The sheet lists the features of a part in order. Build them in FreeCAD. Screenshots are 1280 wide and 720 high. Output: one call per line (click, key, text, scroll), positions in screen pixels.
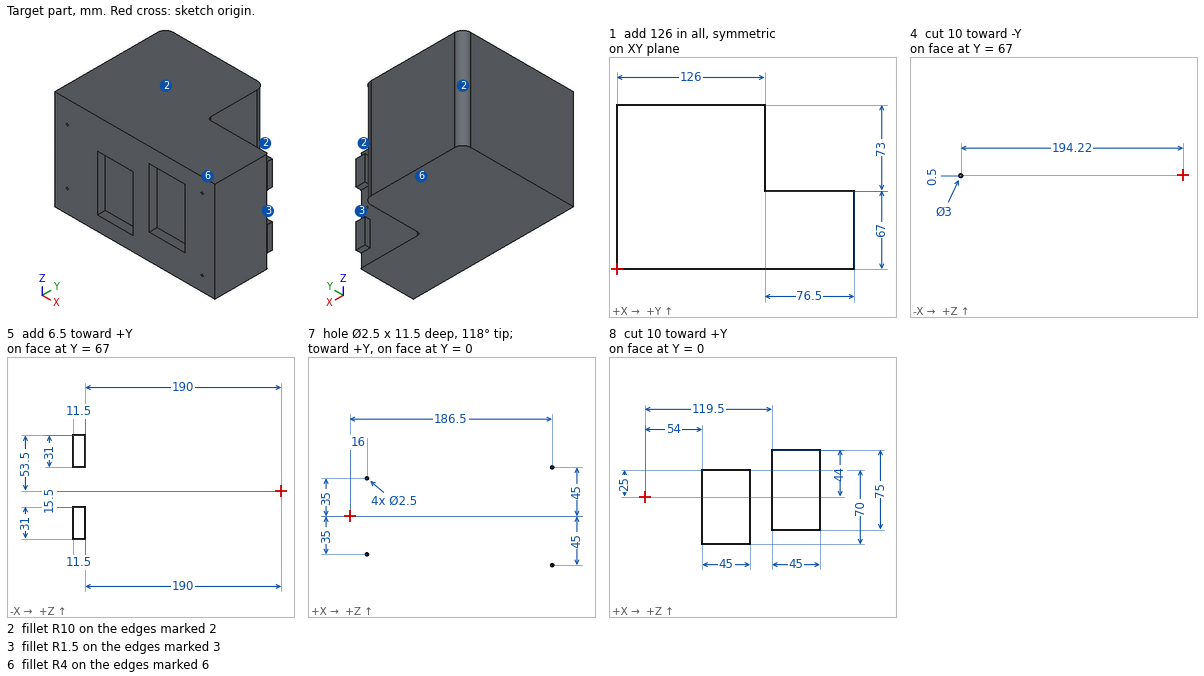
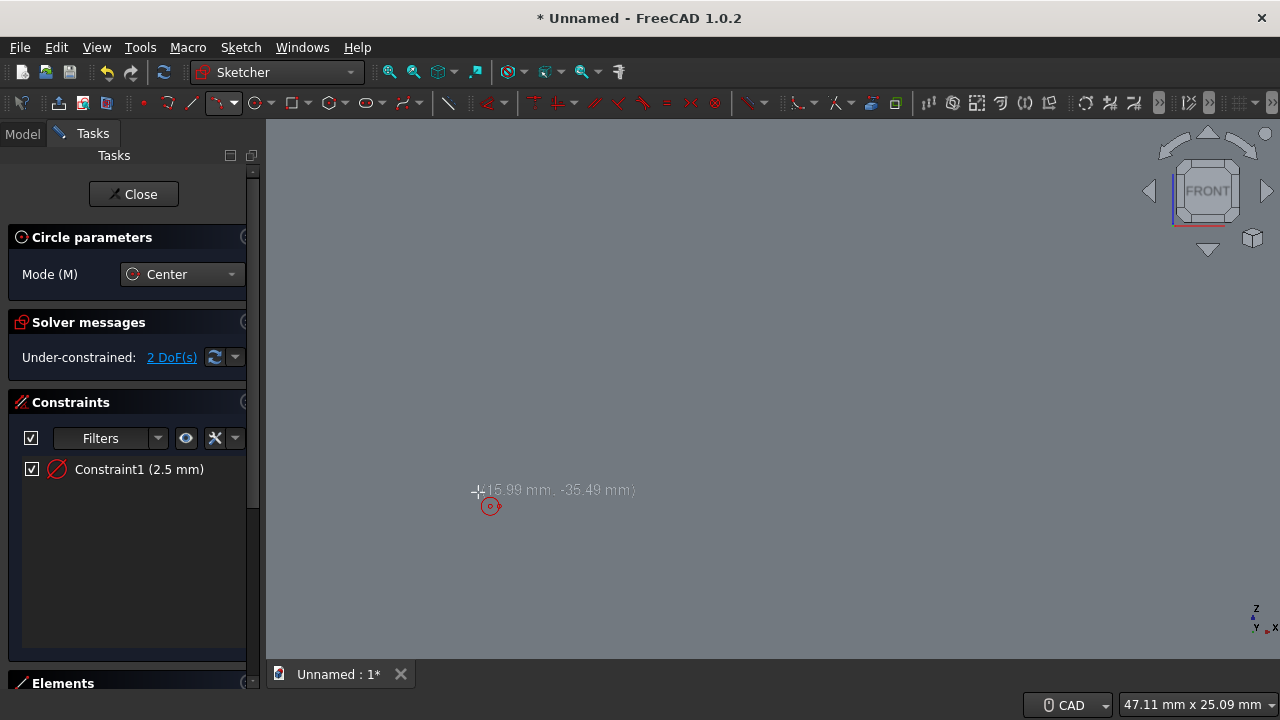
scroll(478, 492, down, 10)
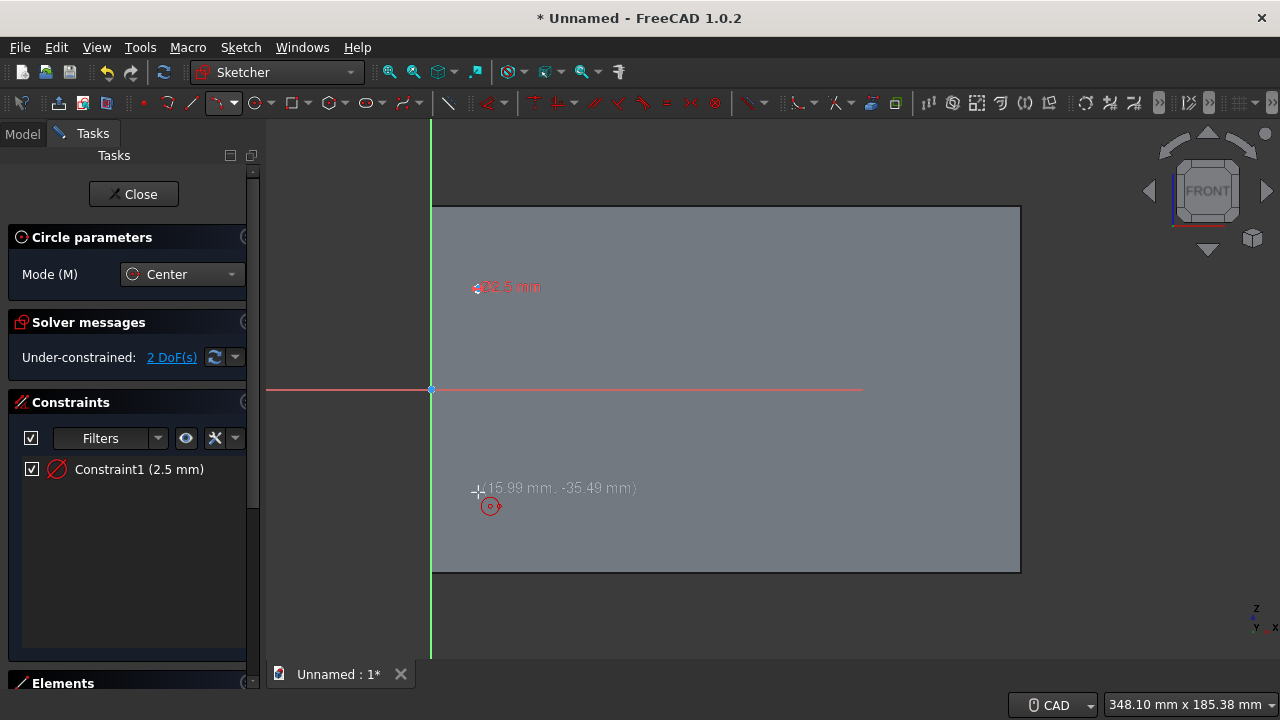
click(478, 492)
move(481, 489)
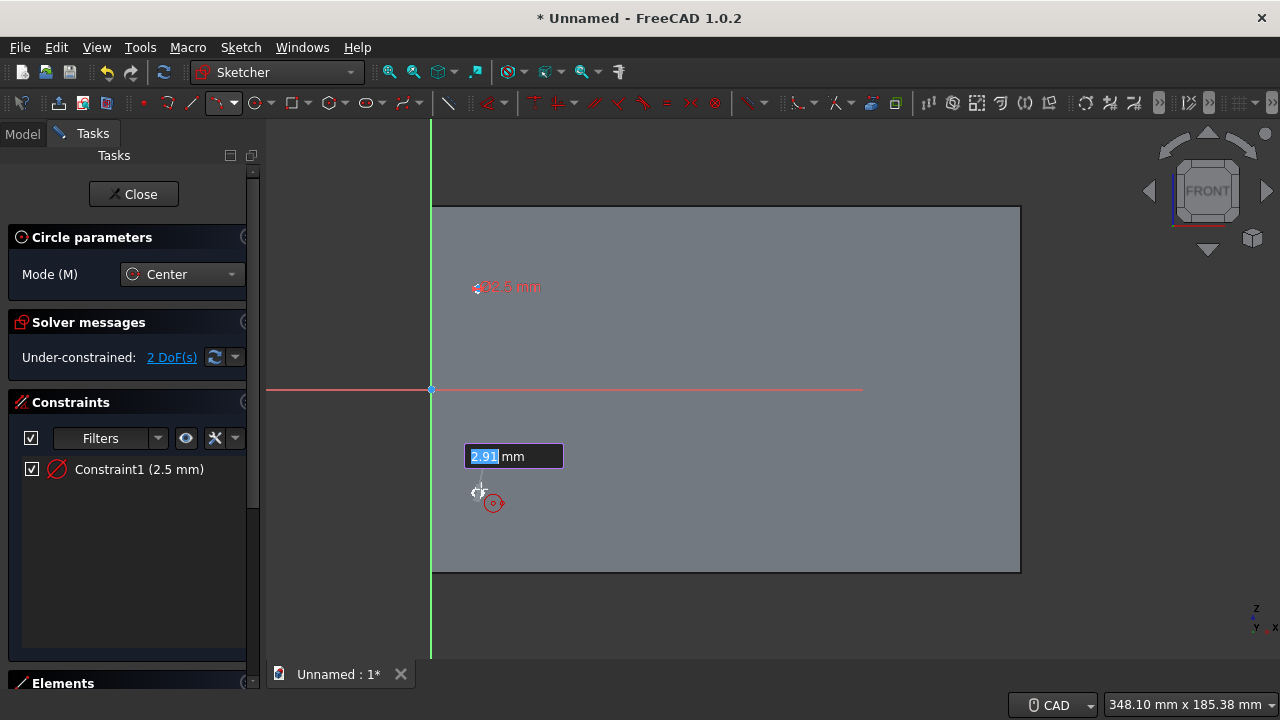
text(2.5)
key(Return)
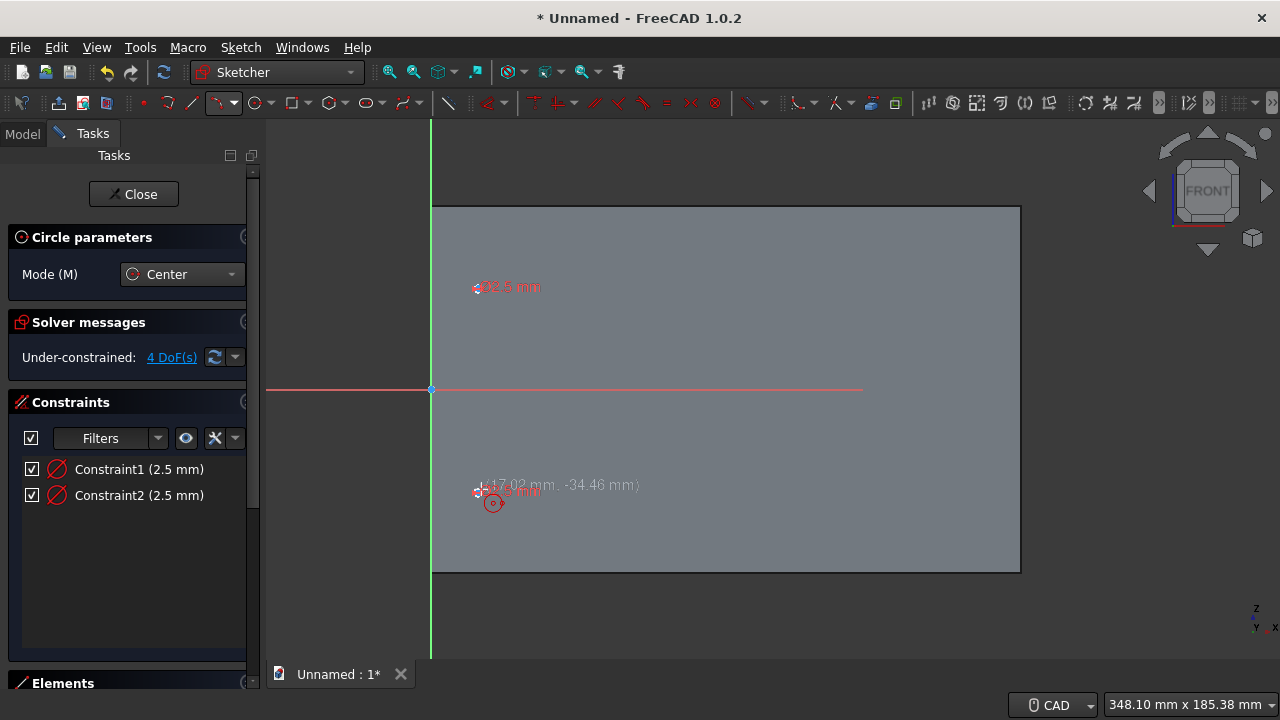
scroll(975, 259, up, 10)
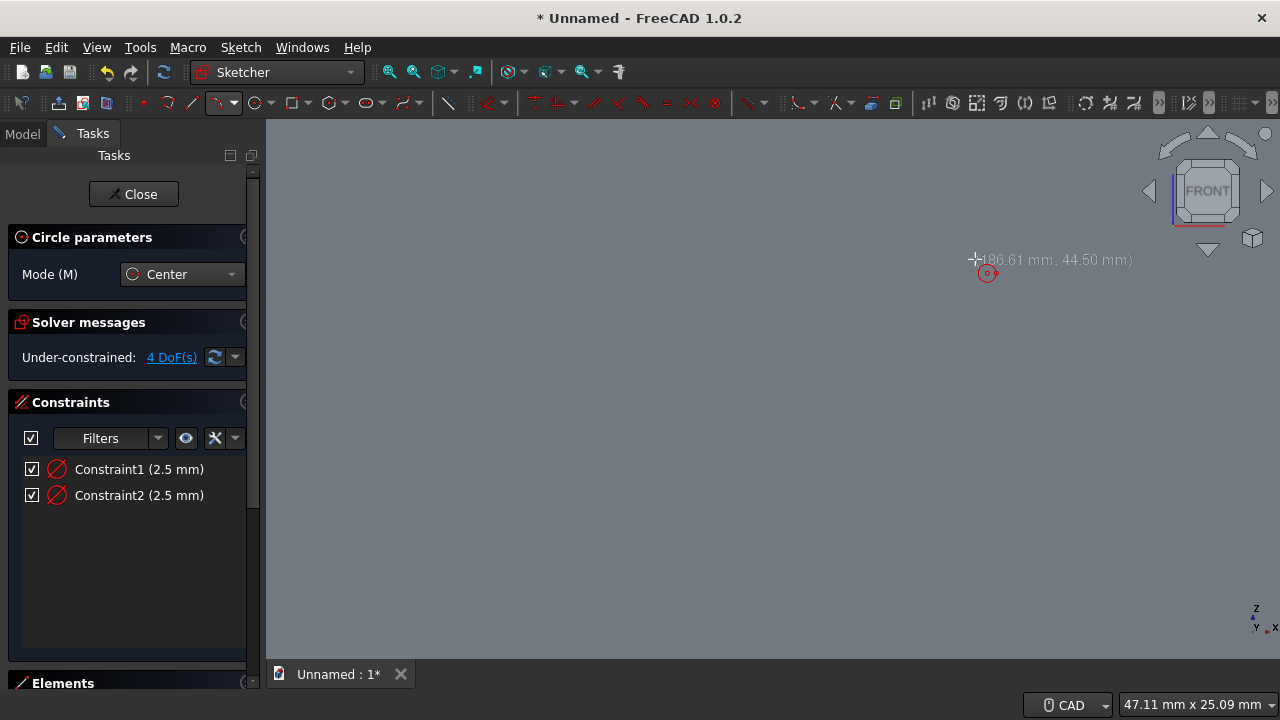
scroll(975, 259, down, 10)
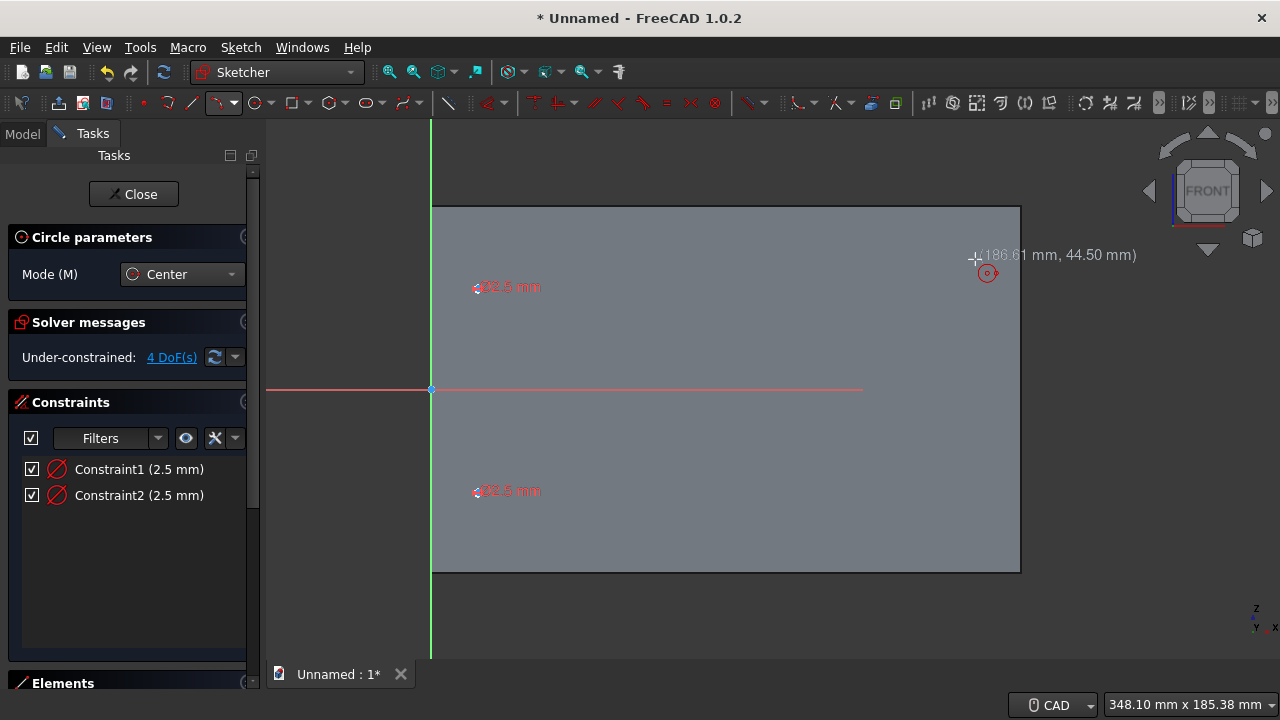
click(975, 259)
move(977, 256)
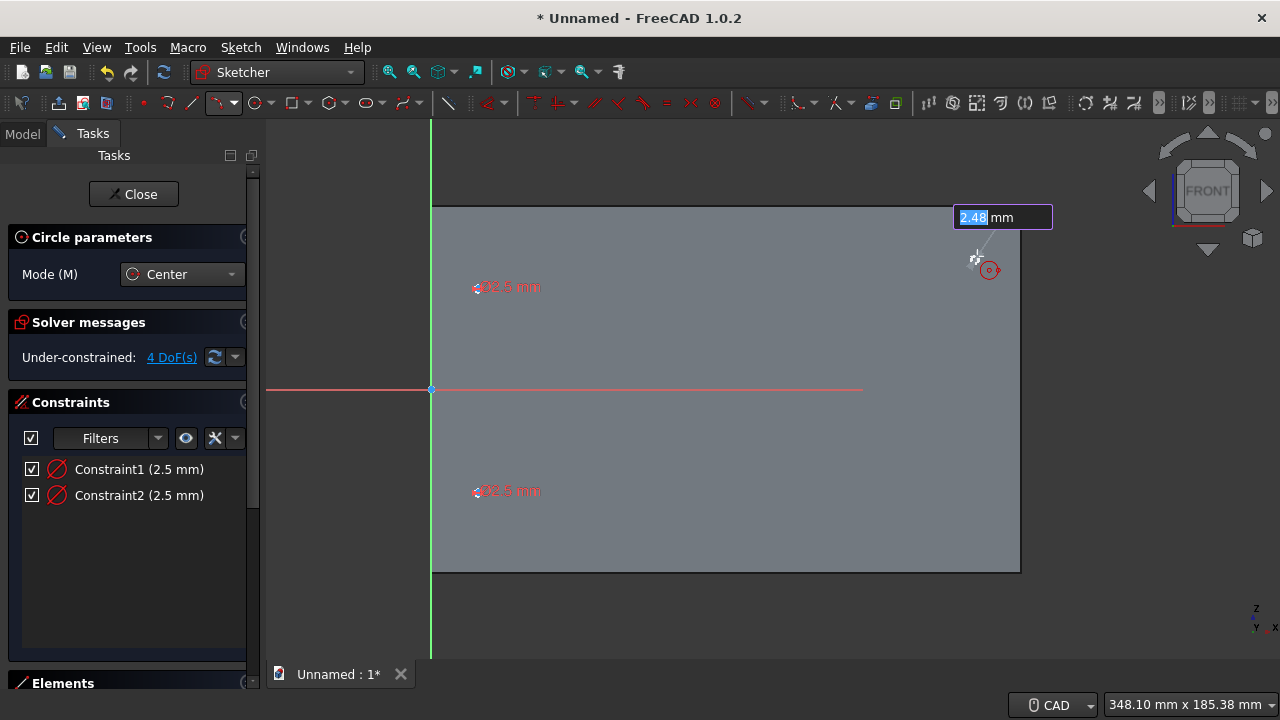
text(2.5)
key(Return)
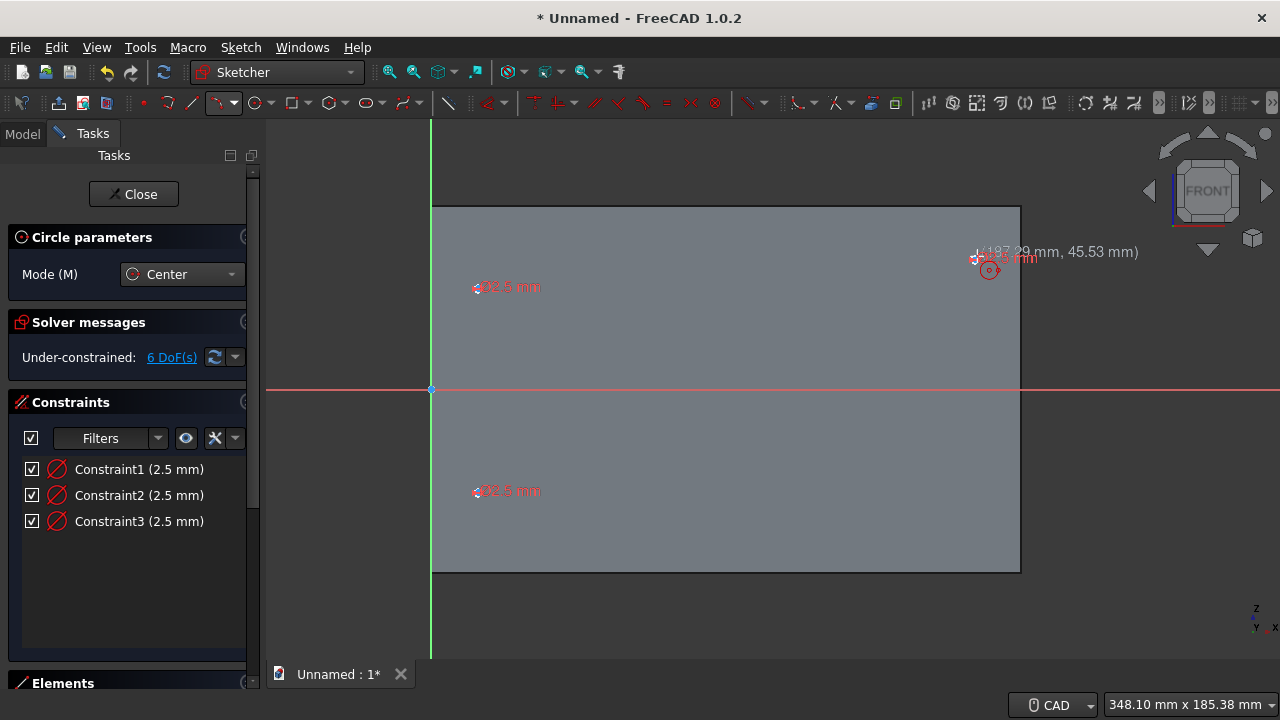
scroll(975, 521, up, 10)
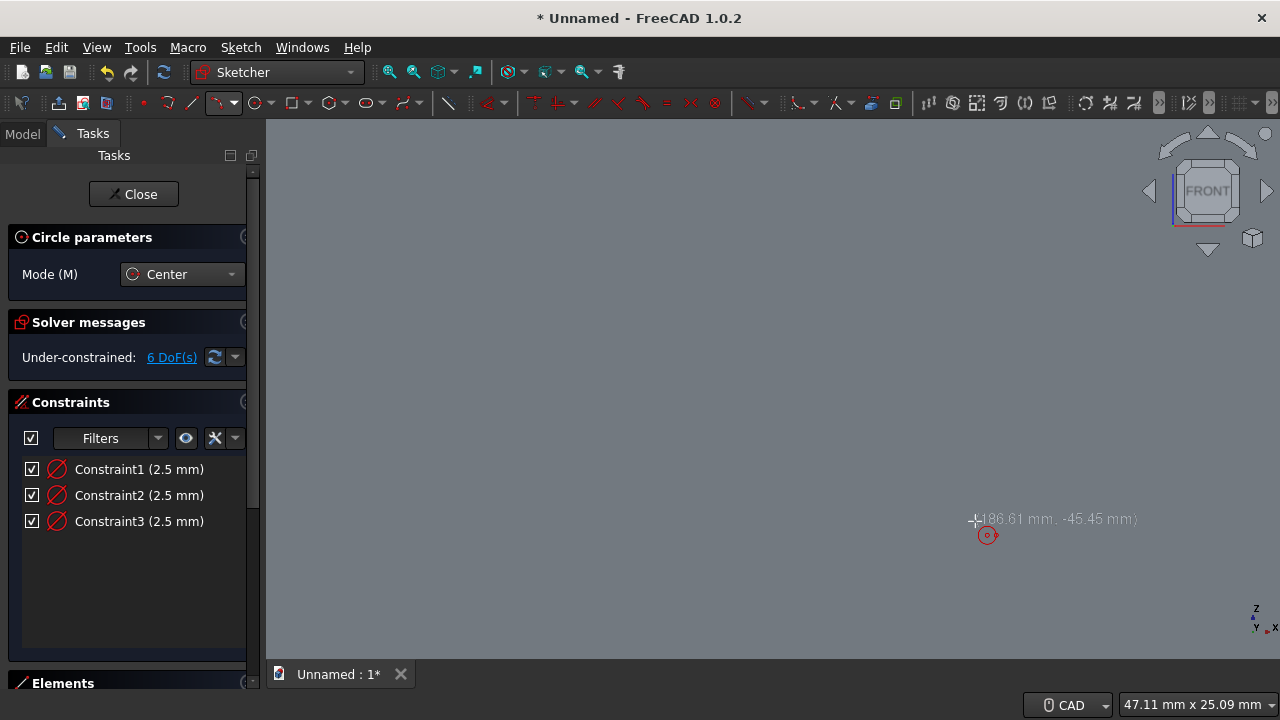
scroll(975, 521, down, 10)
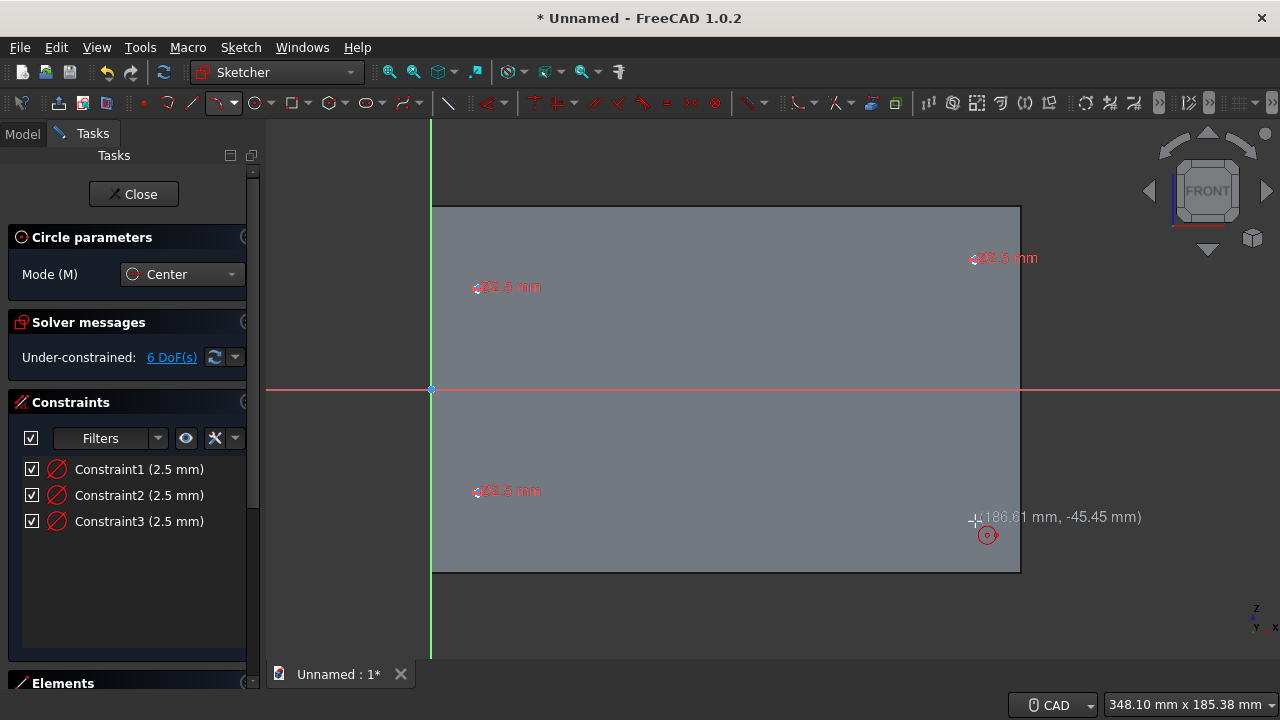
click(975, 521)
move(977, 518)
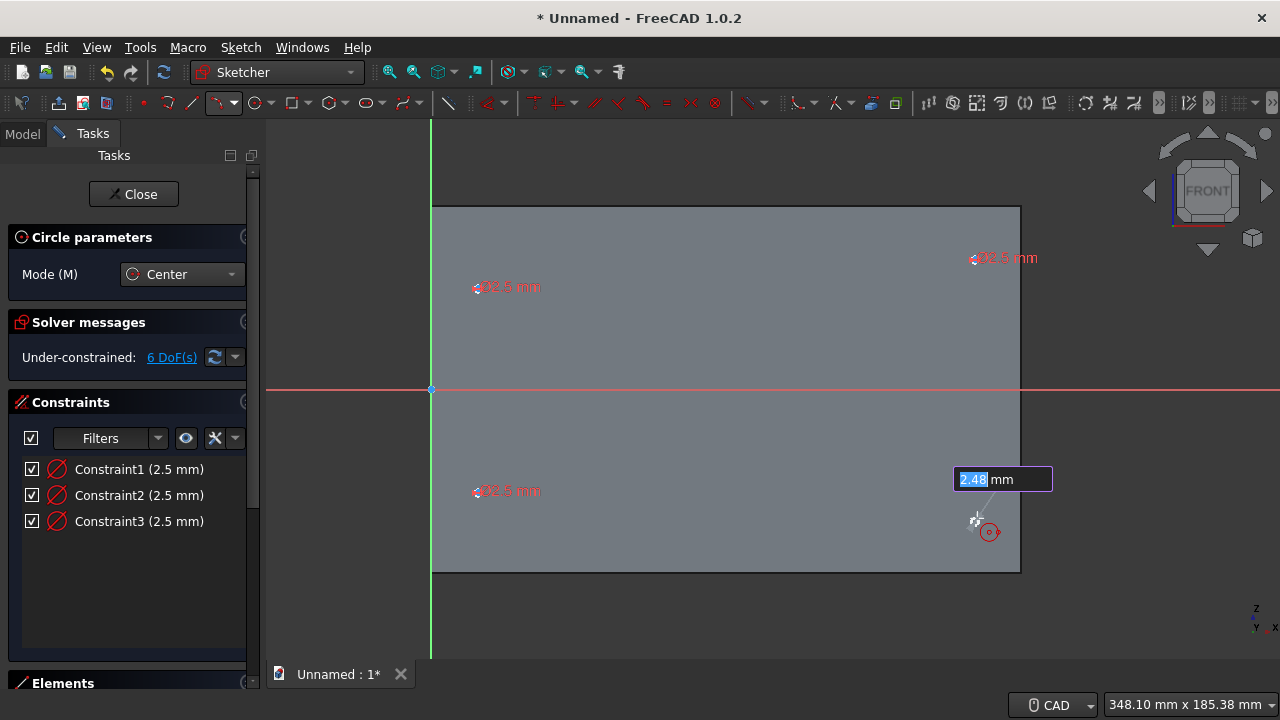
text(2.5)
key(Return)
key(Escape)